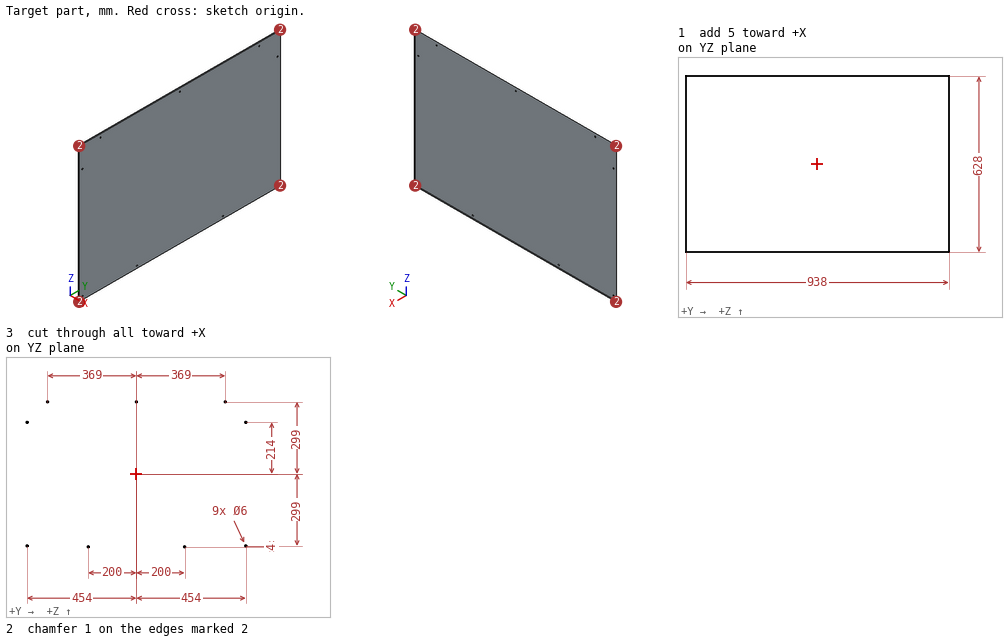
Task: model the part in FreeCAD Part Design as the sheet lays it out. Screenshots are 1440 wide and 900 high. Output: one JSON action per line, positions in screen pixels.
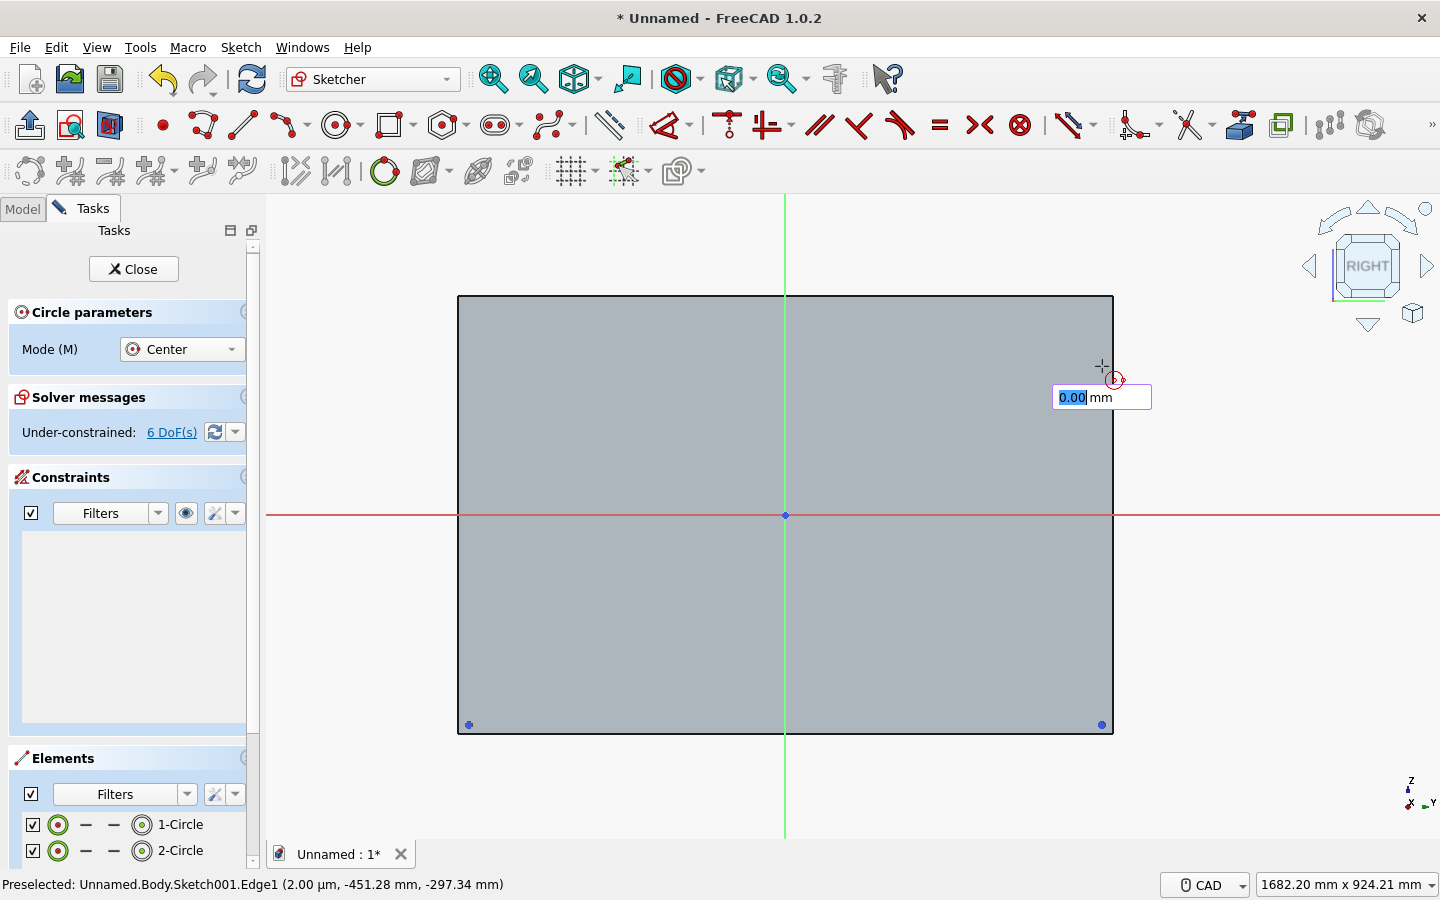
{"action": "scroll", "coordinate": [1104, 364], "scroll_direction": "up", "scroll_amount": 11}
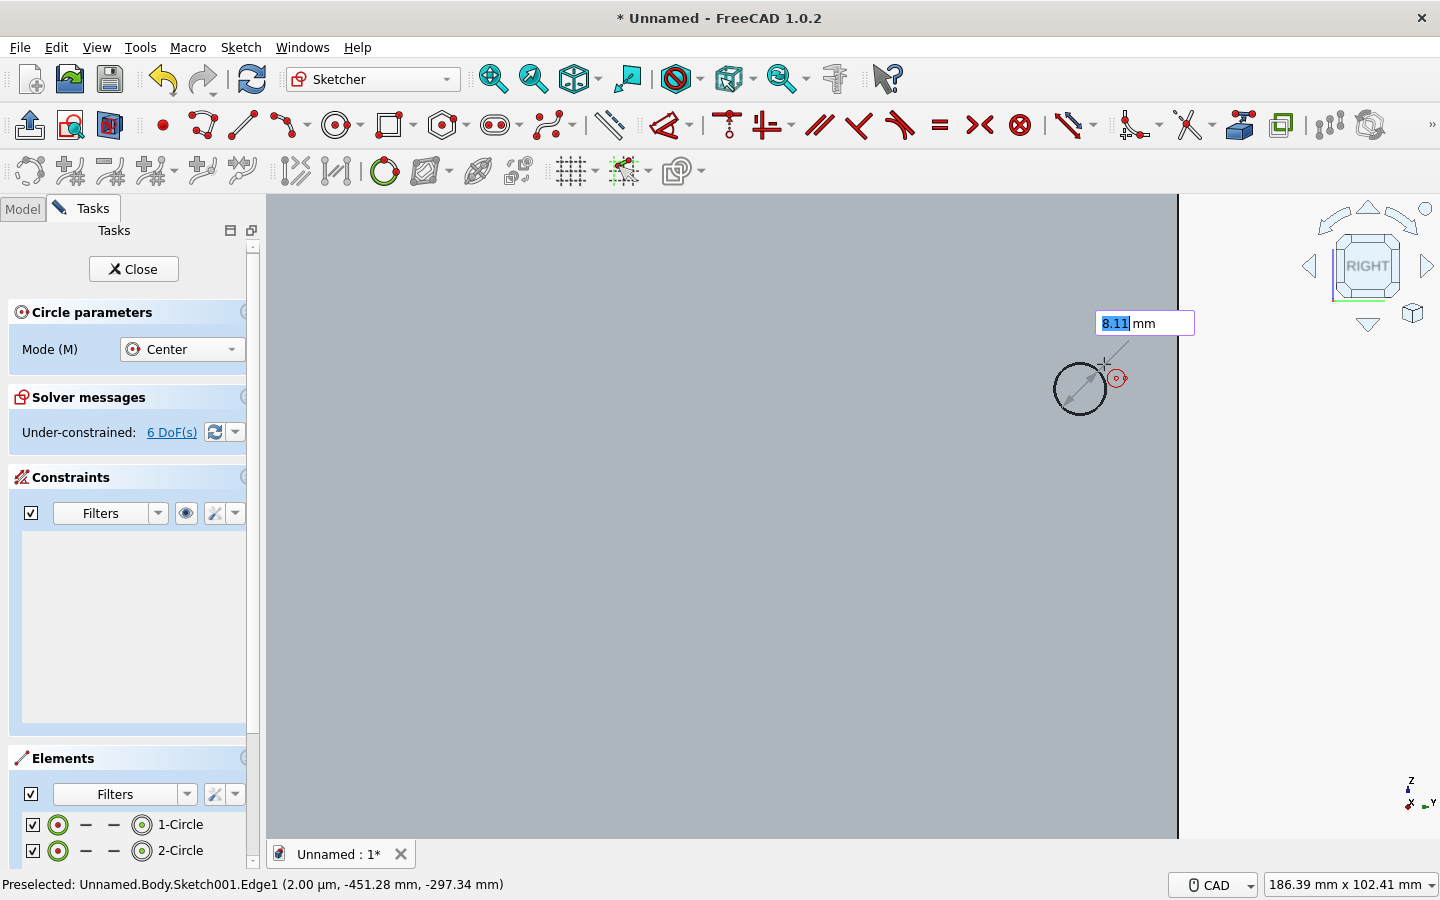
{"action": "left_click", "coordinate": [1097, 363]}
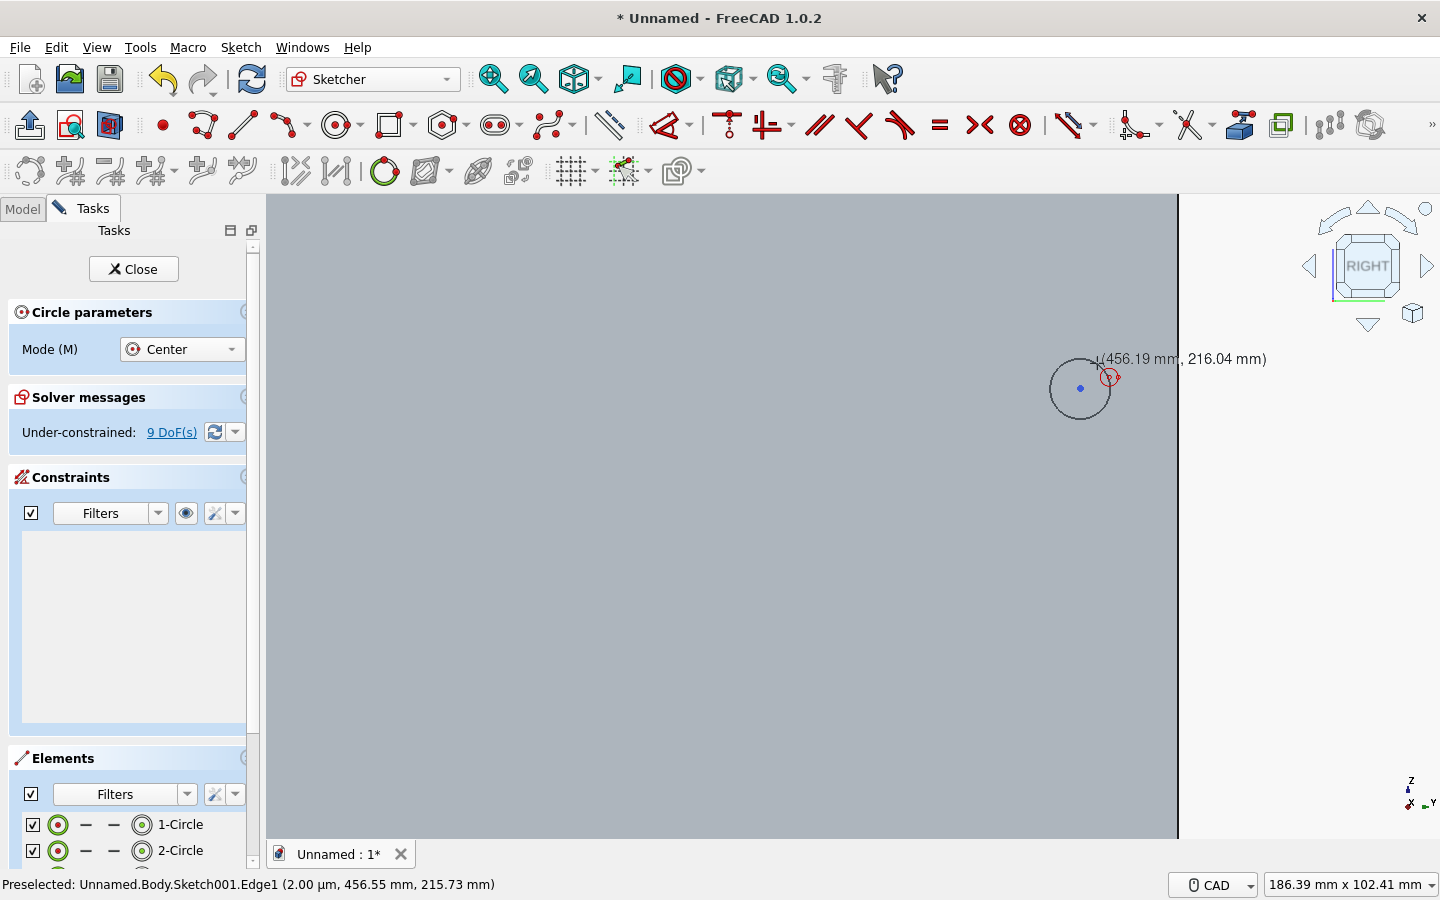
{"action": "scroll", "coordinate": [1104, 364], "scroll_direction": "down", "scroll_amount": 11}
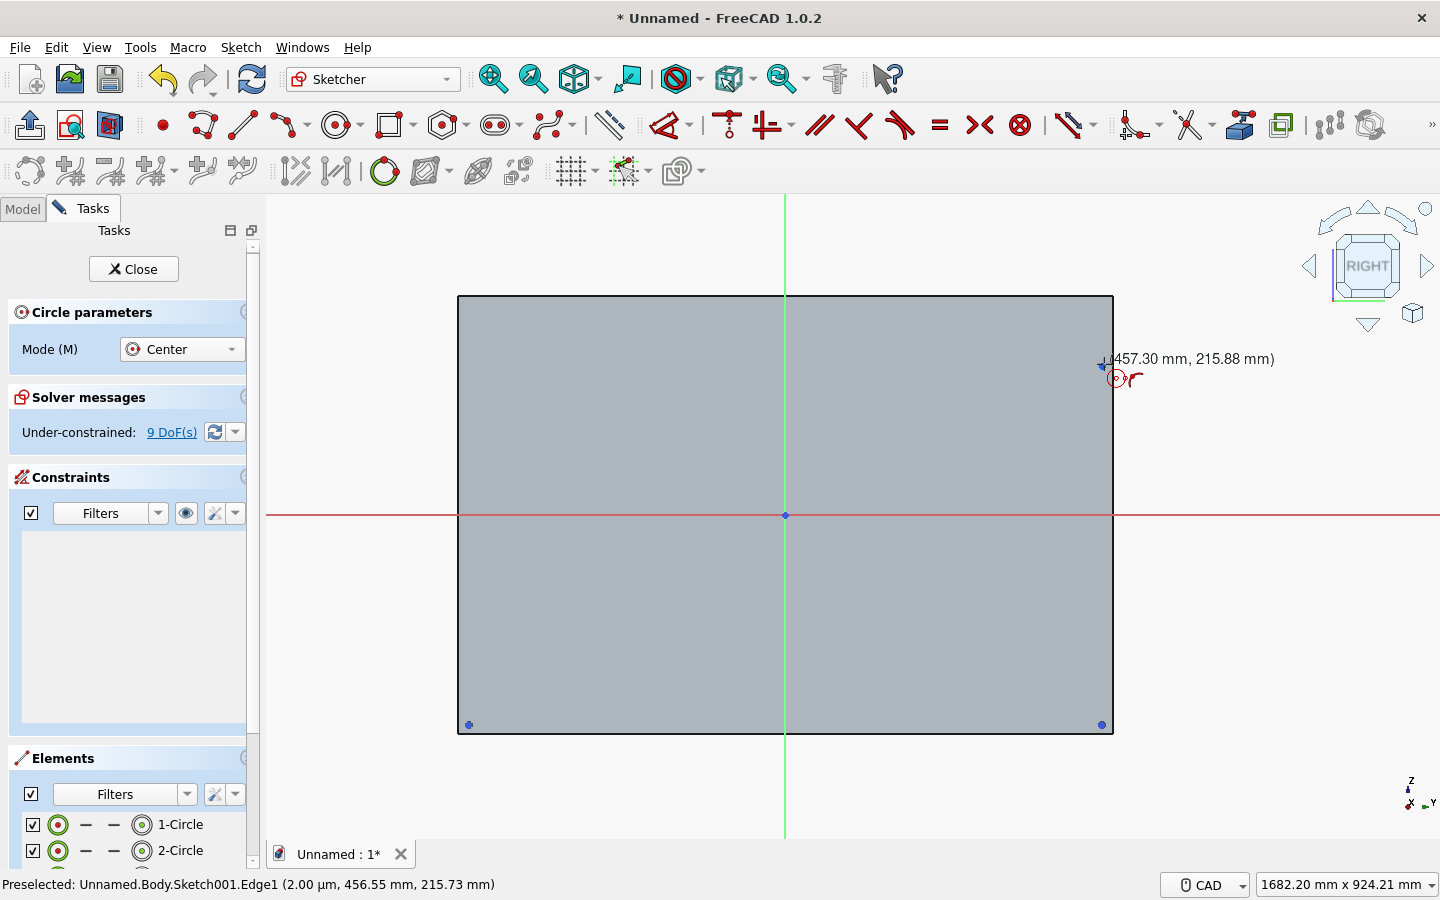
{"action": "scroll", "coordinate": [1043, 306], "scroll_direction": "up", "scroll_amount": 12}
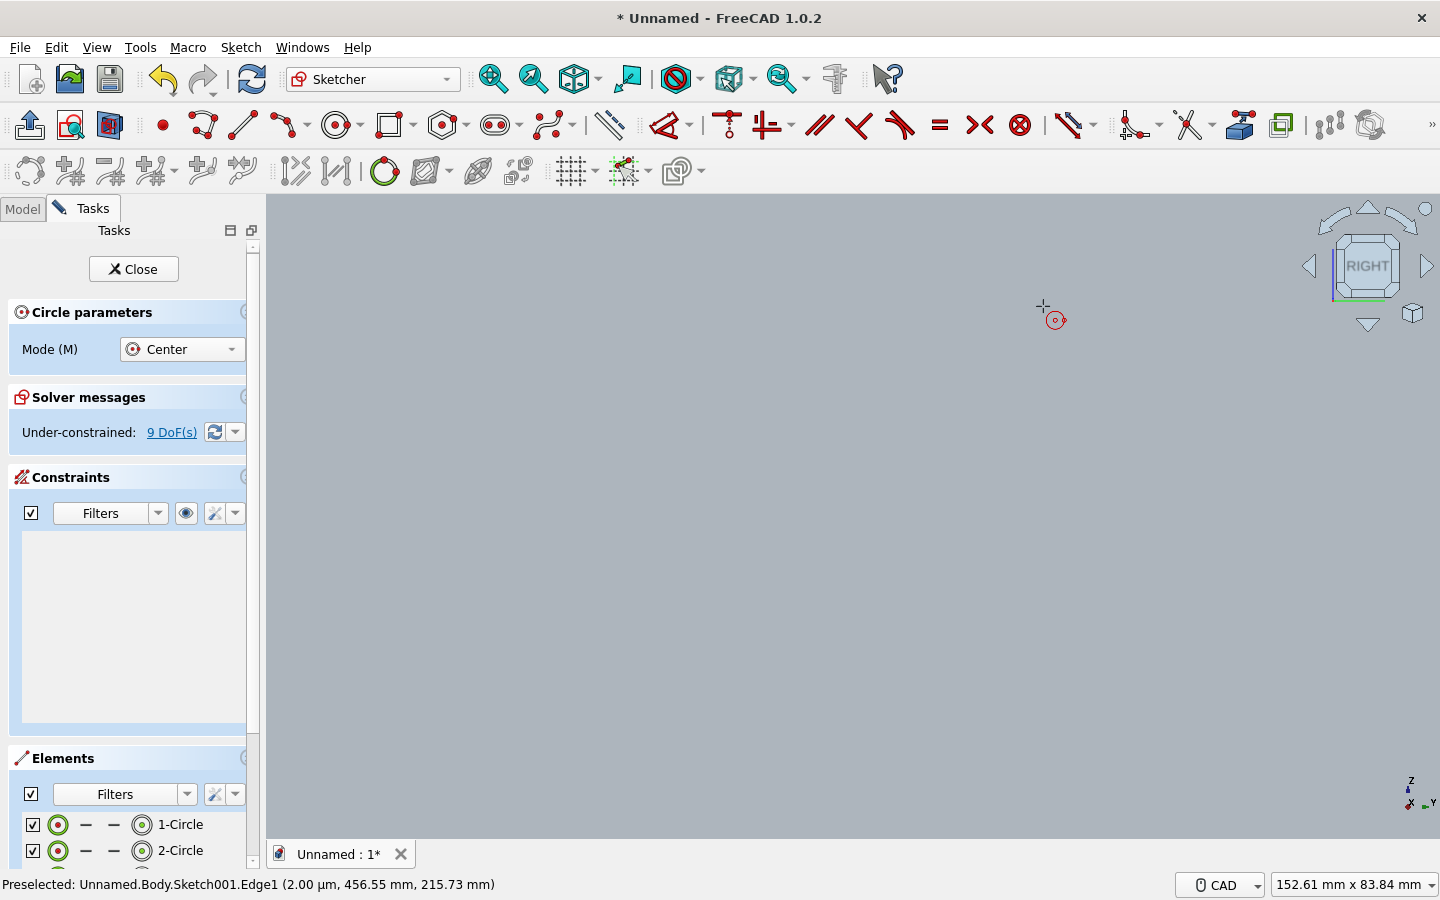
{"action": "scroll", "coordinate": [1043, 306], "scroll_direction": "down", "scroll_amount": 12}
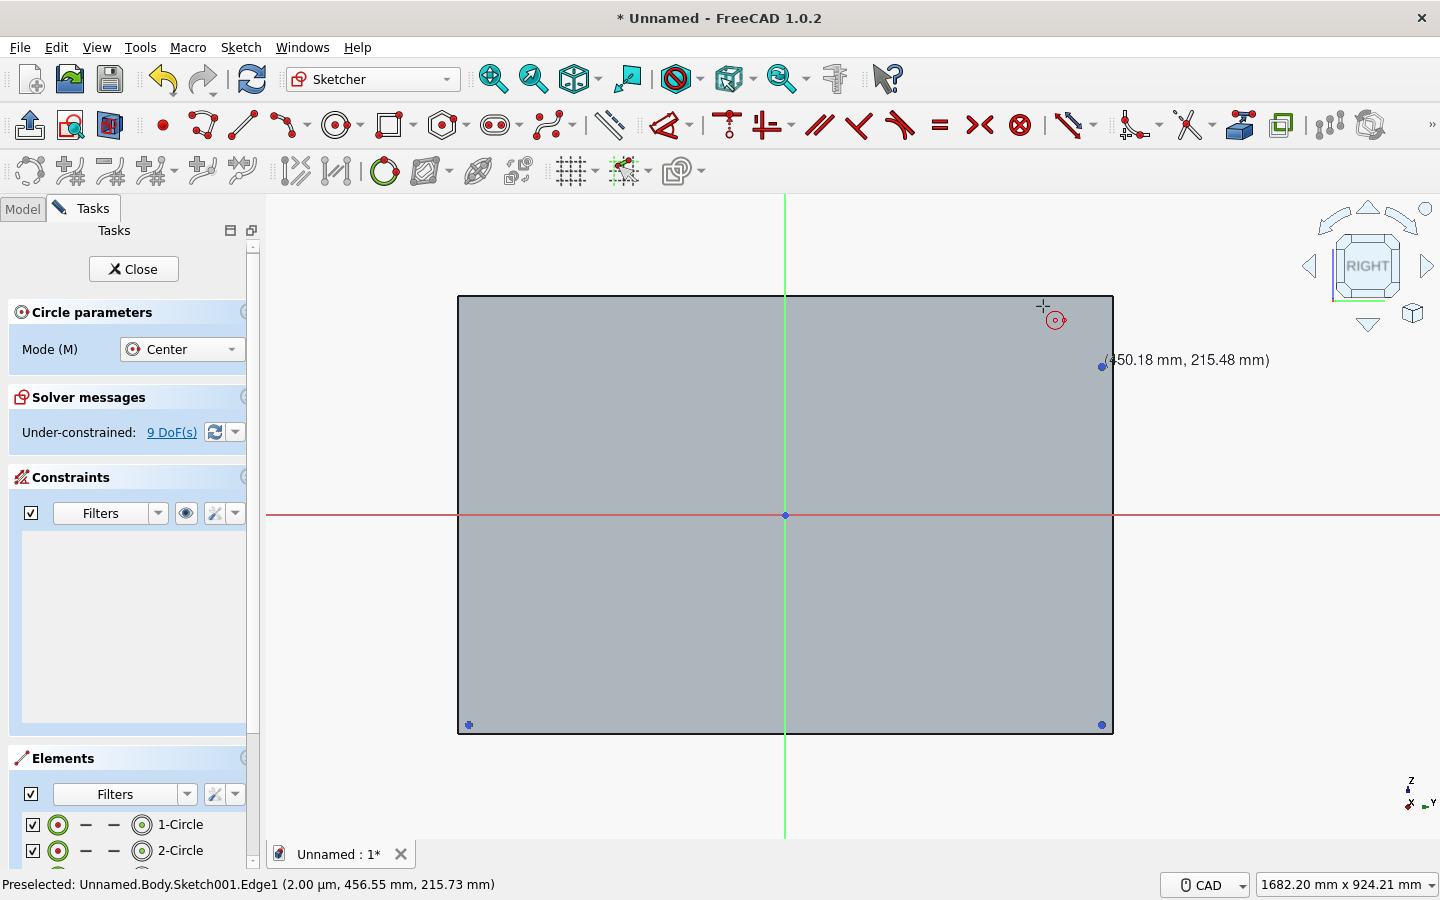
{"action": "left_click", "coordinate": [1043, 306]}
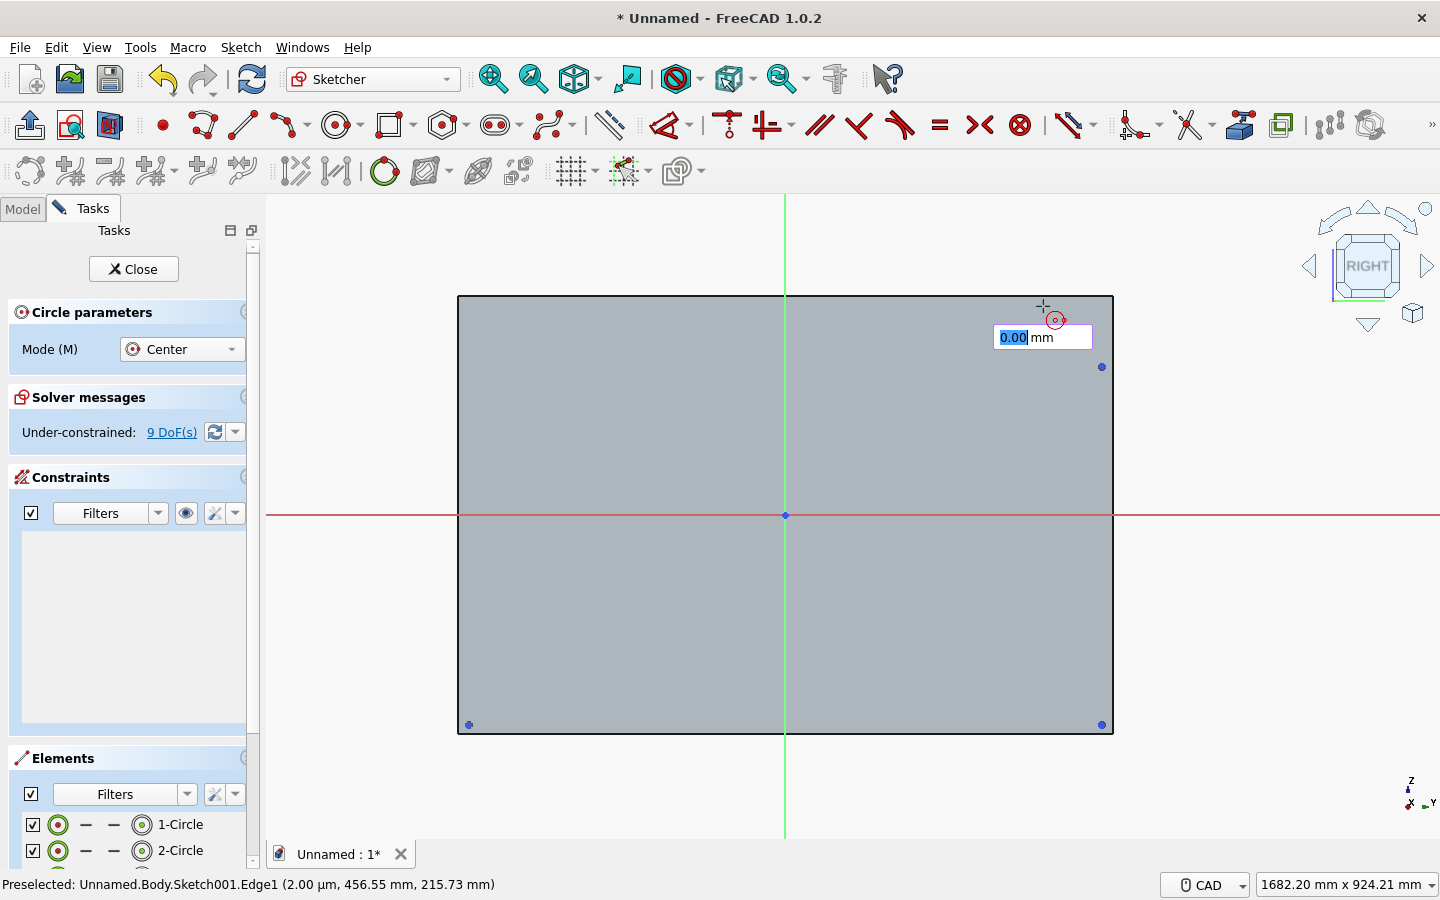
{"action": "scroll", "coordinate": [1044, 305], "scroll_direction": "up", "scroll_amount": 11}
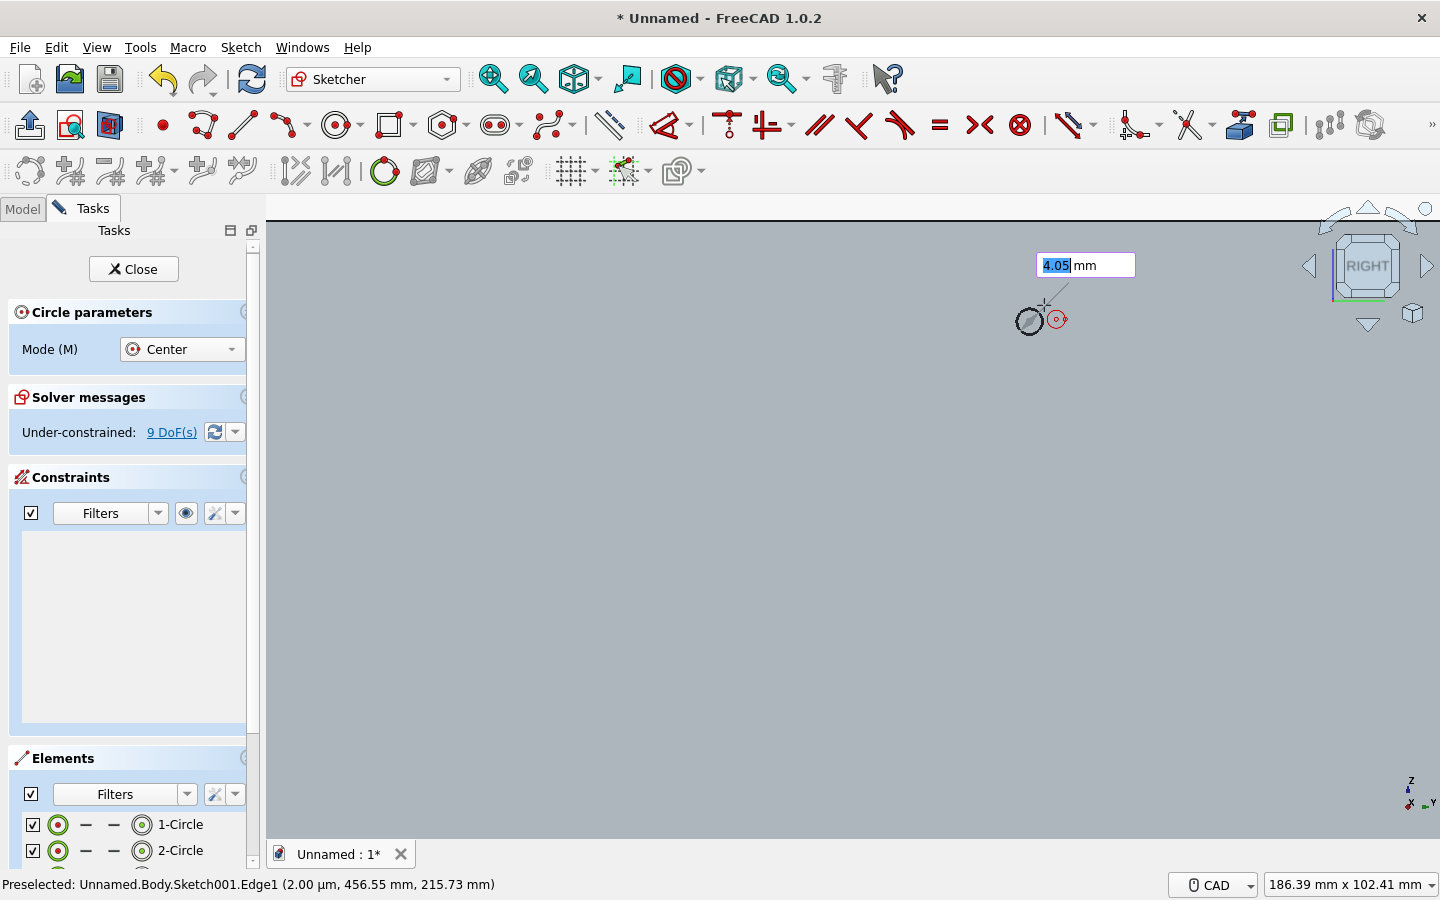
{"action": "left_click", "coordinate": [1043, 302]}